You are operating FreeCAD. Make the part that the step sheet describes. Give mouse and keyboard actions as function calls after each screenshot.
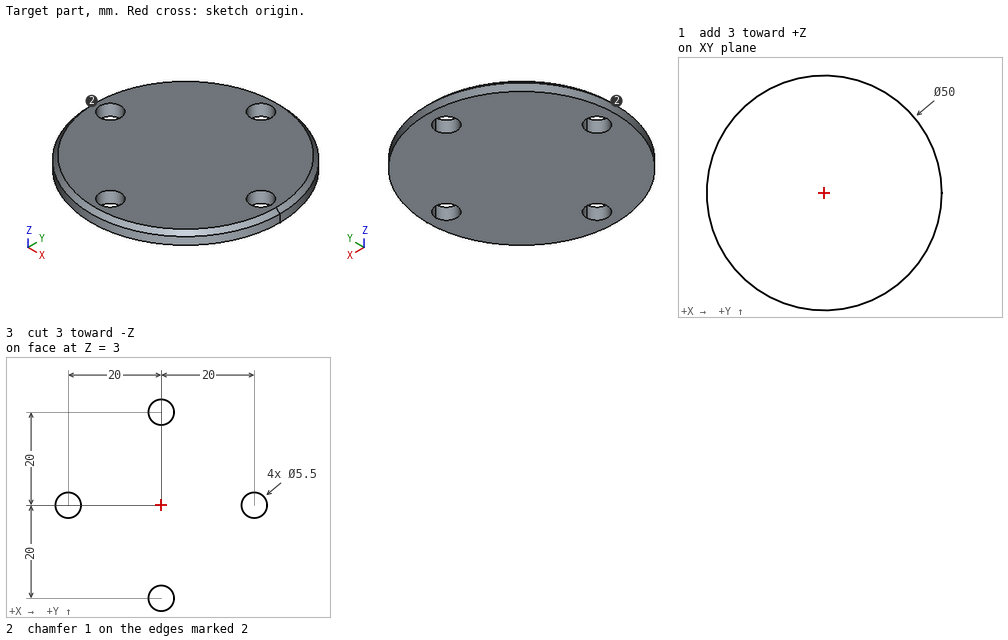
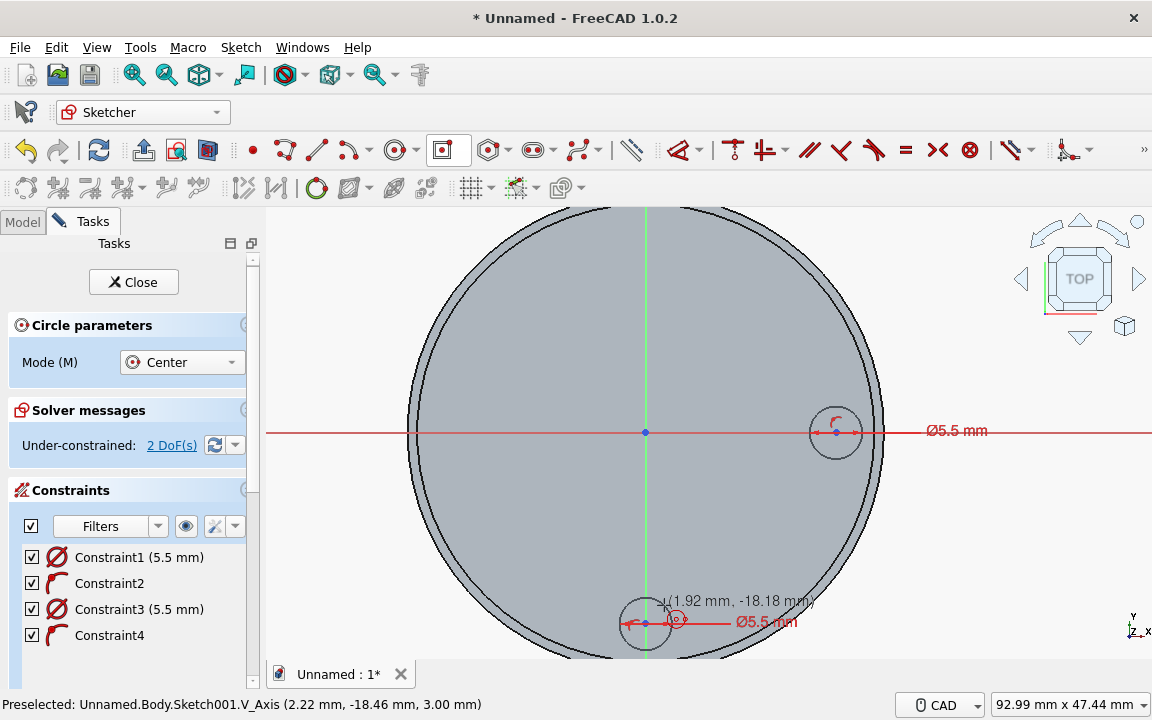
click(455, 433)
move(474, 414)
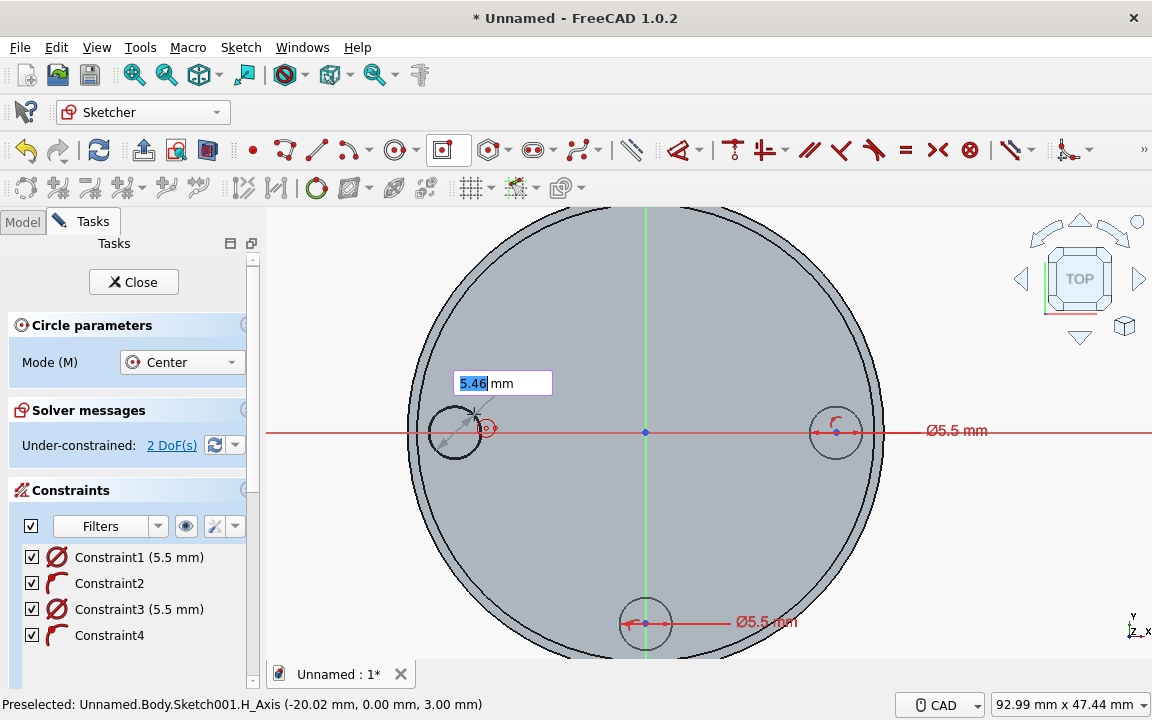
text(5.5)
key(Return)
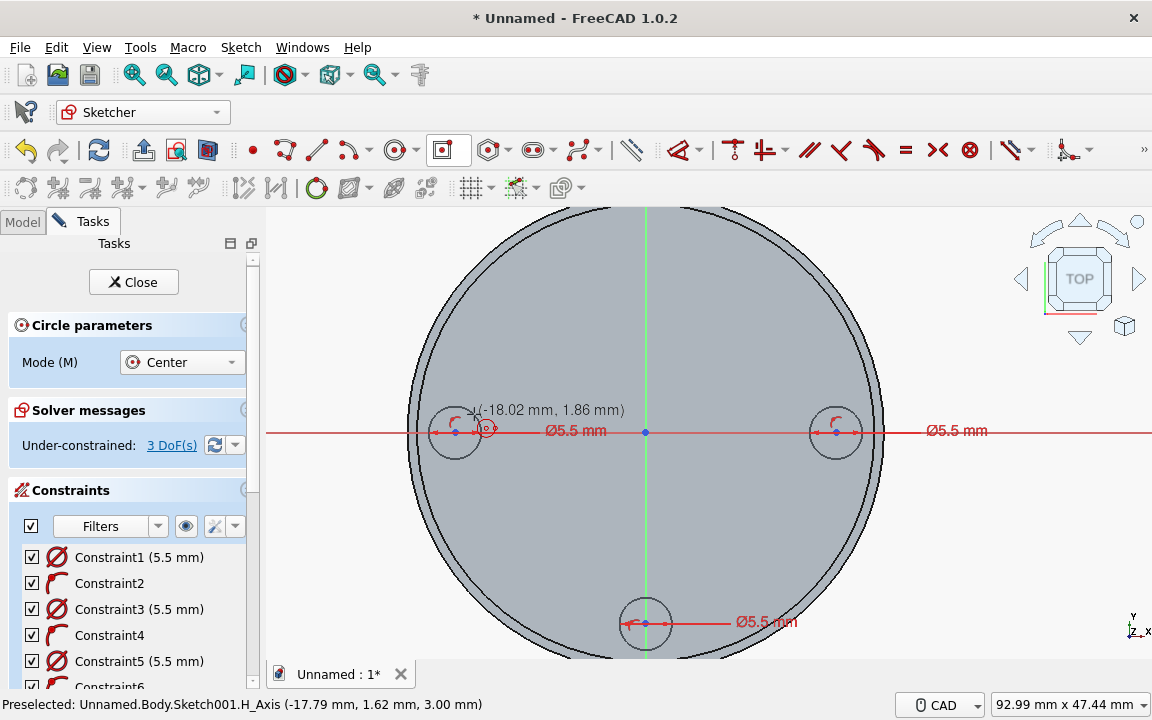
click(646, 242)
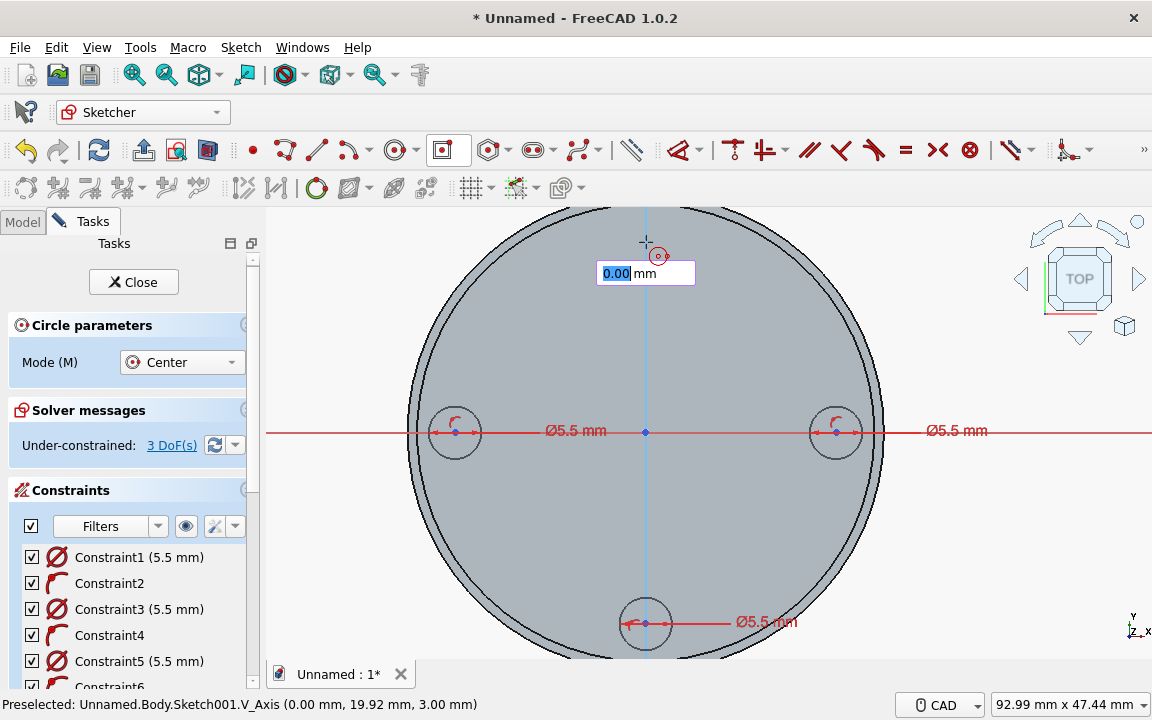
scroll(630, 434, down, 2)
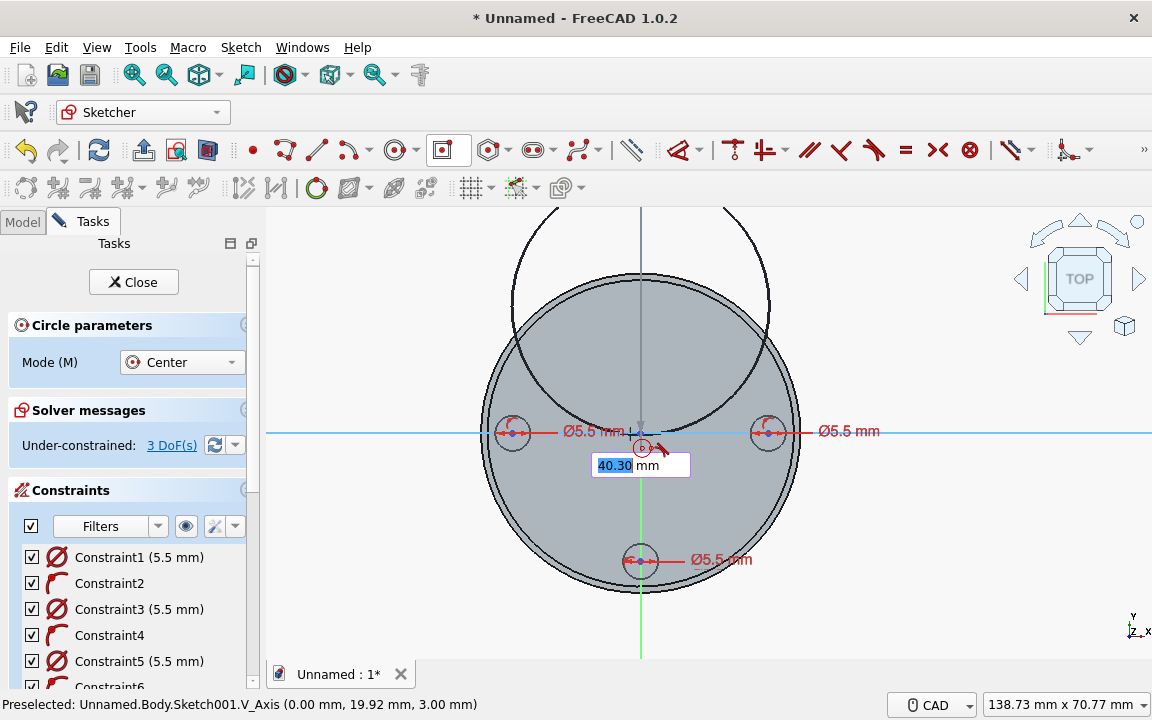
scroll(653, 293, up, 2)
move(653, 293)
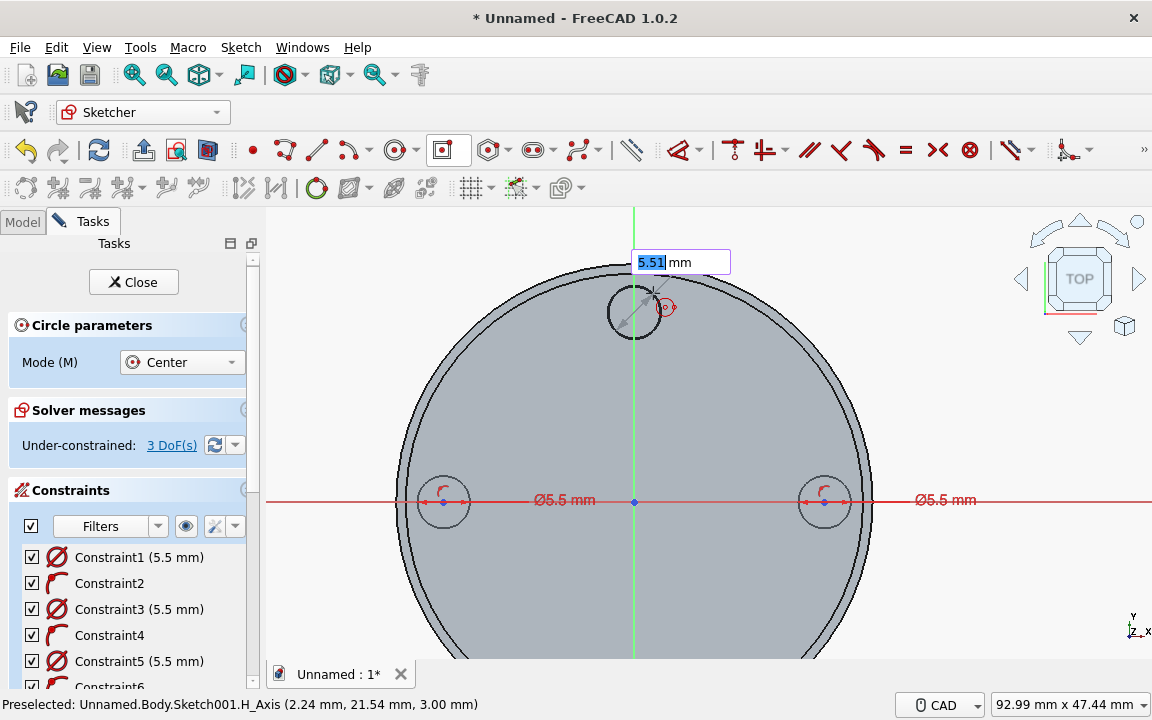
text(5.5)
key(Return)
key(Escape)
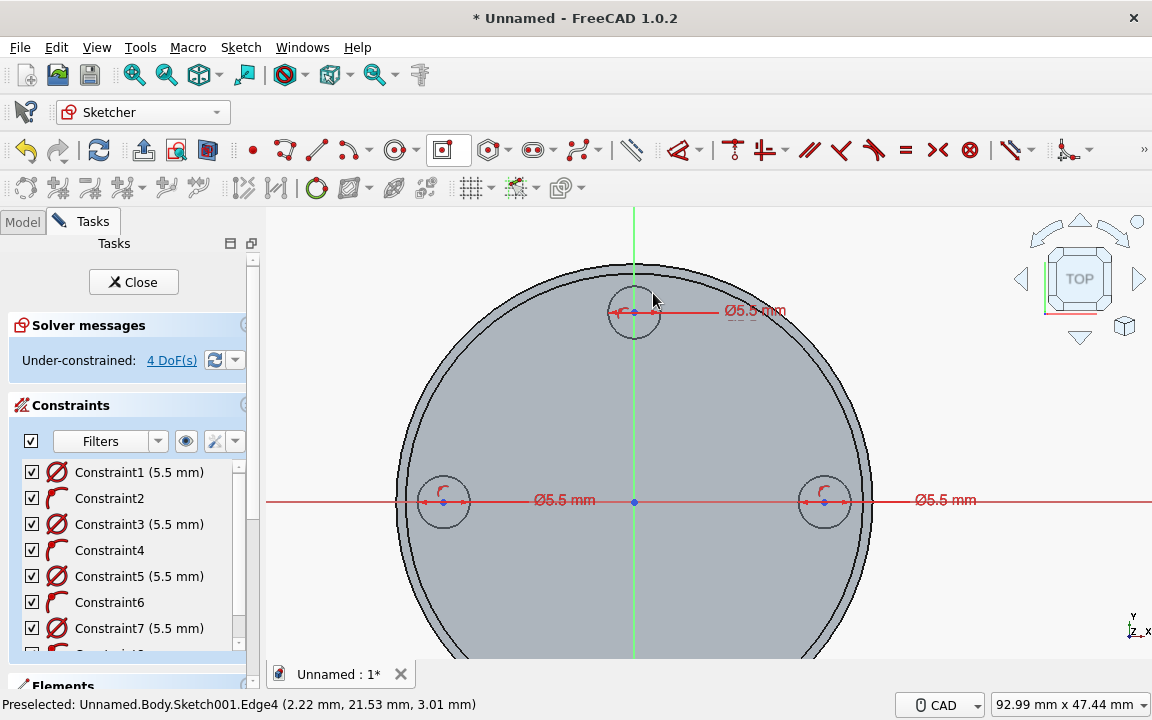
click(825, 502)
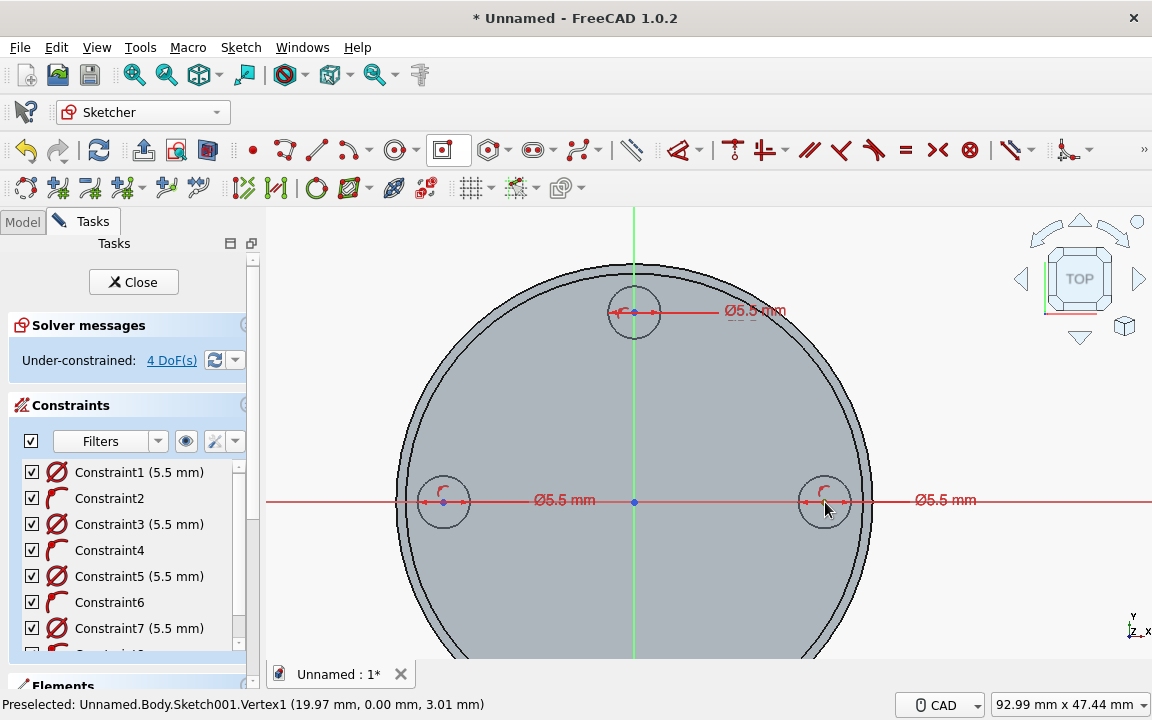
key(l)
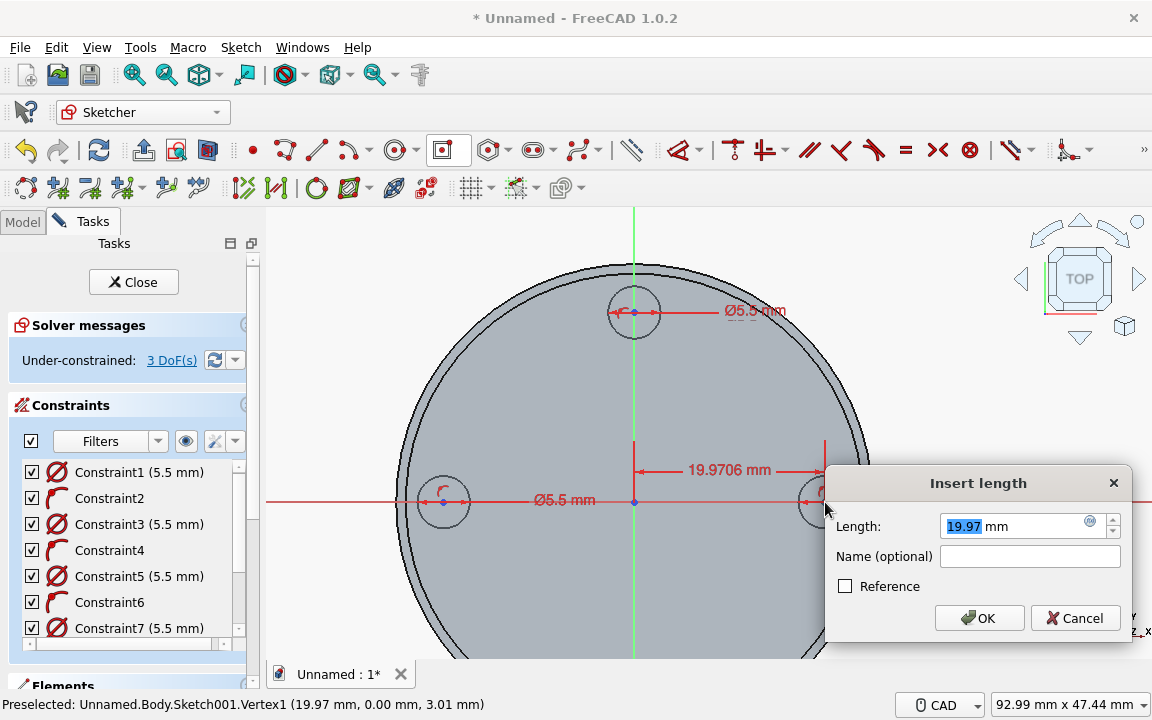
text(20)
key(Return)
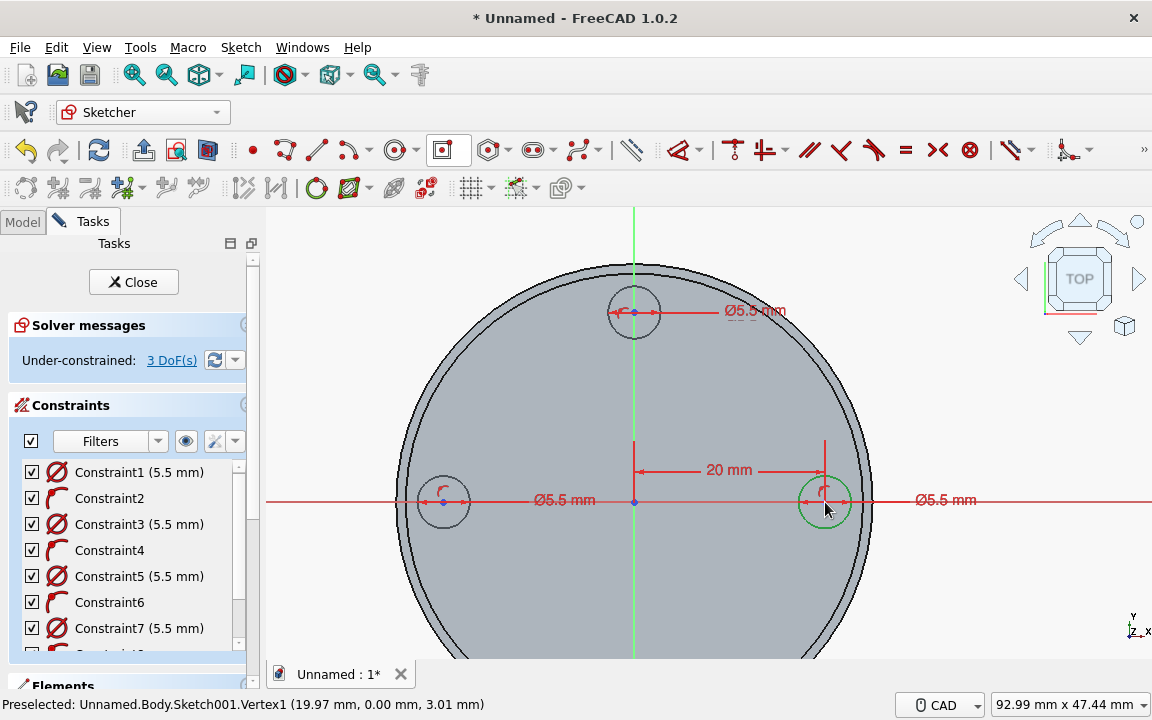
scroll(653, 292, down, 2)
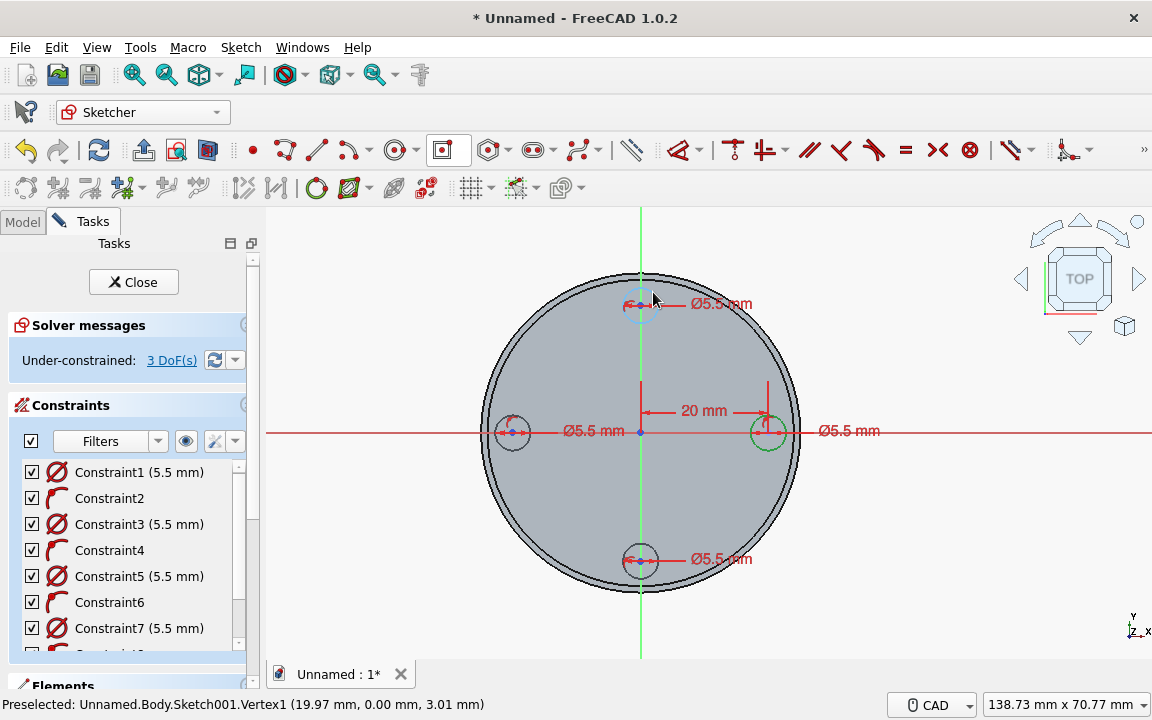
click(641, 561)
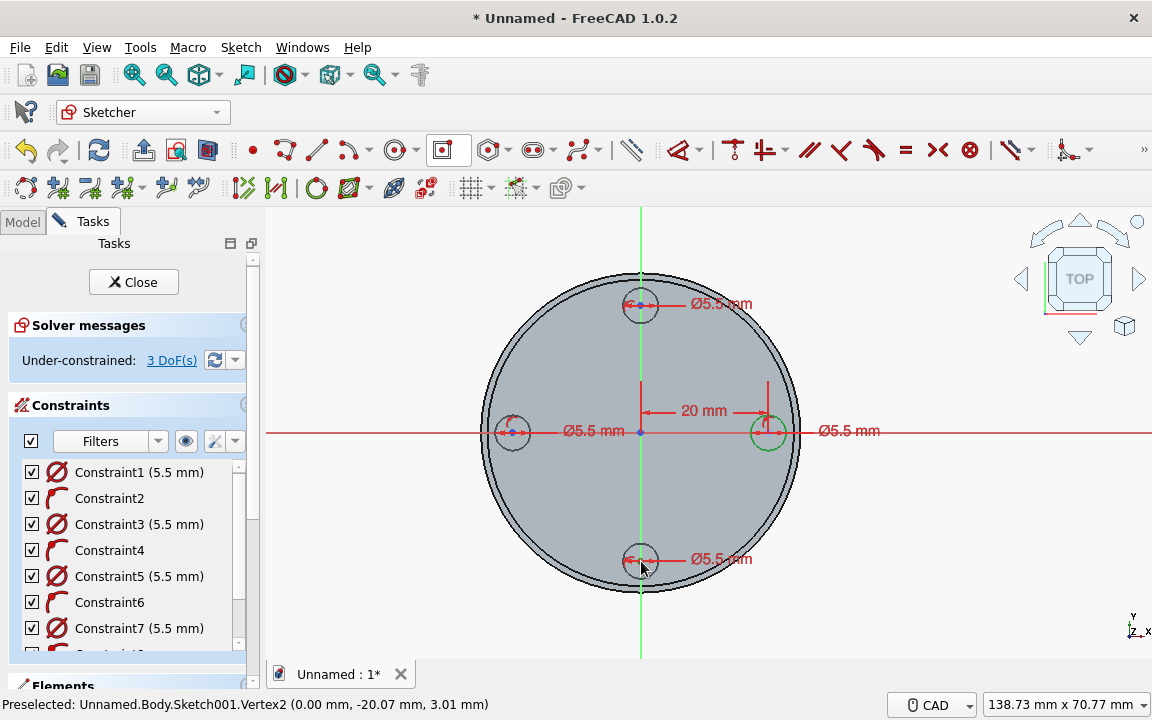
key(i)